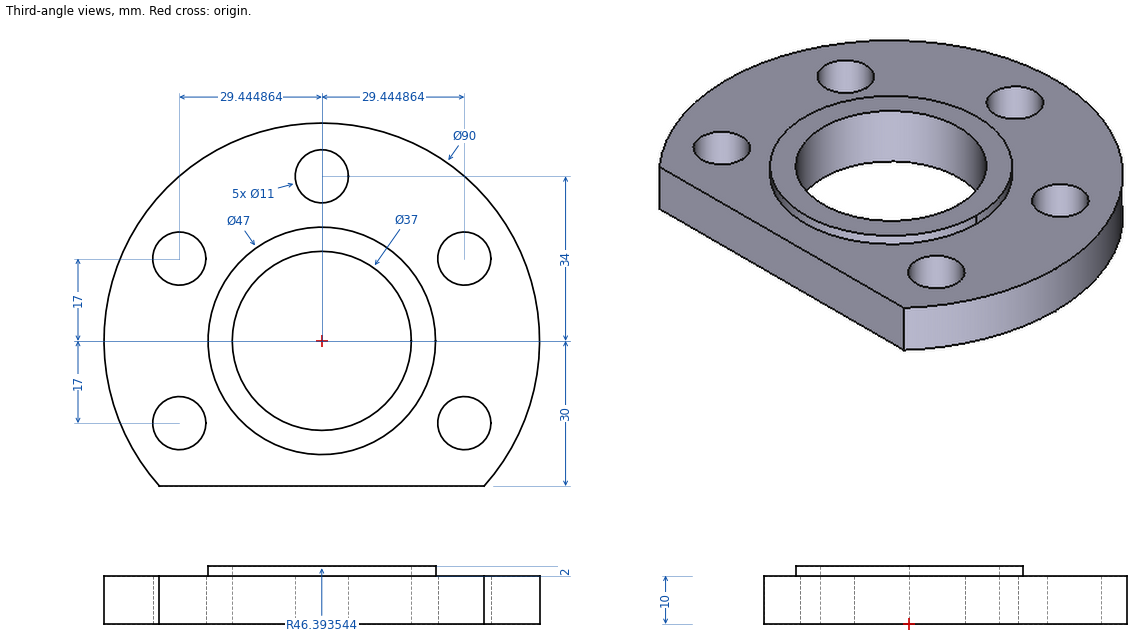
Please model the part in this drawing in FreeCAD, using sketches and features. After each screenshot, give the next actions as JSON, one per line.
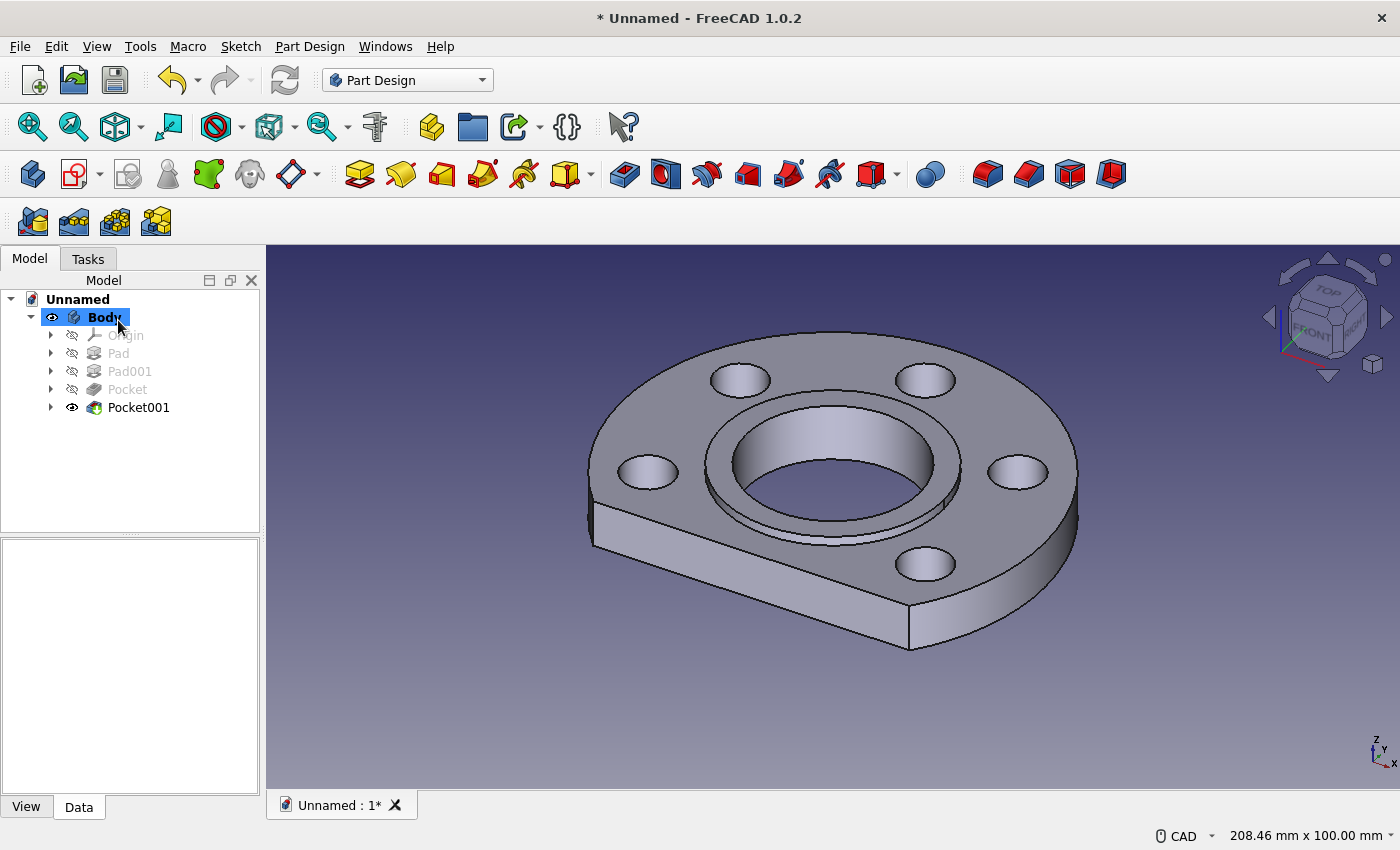
{"action": "key", "text": "0"}